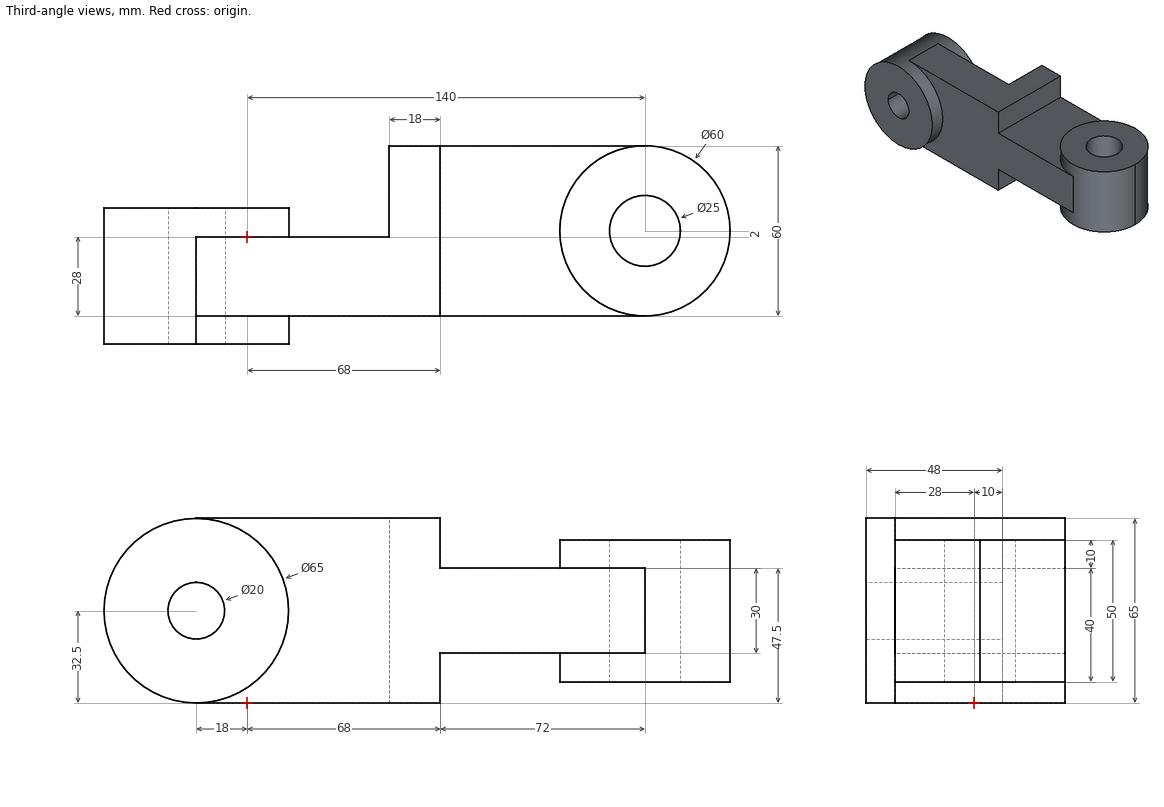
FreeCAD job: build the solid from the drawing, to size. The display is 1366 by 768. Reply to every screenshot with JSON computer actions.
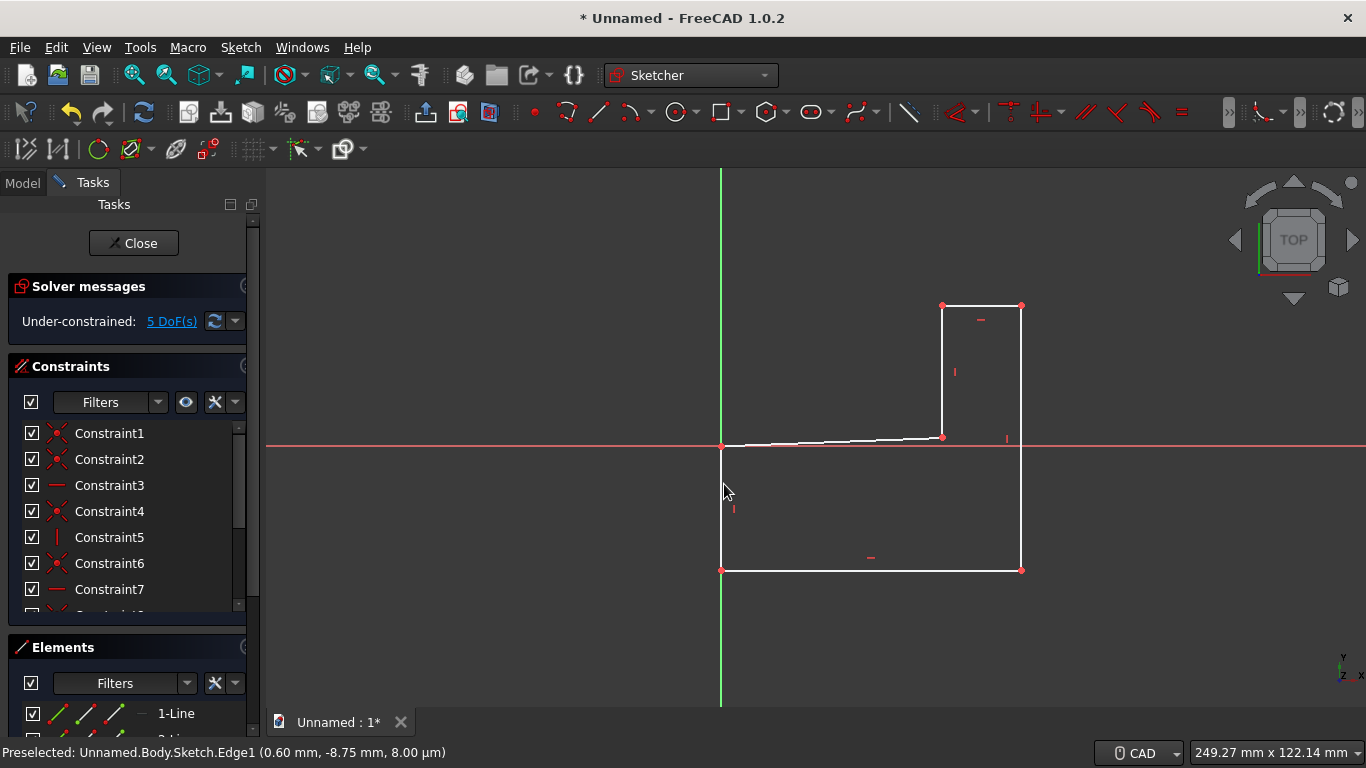
{"action": "left_click", "coordinate": [788, 444]}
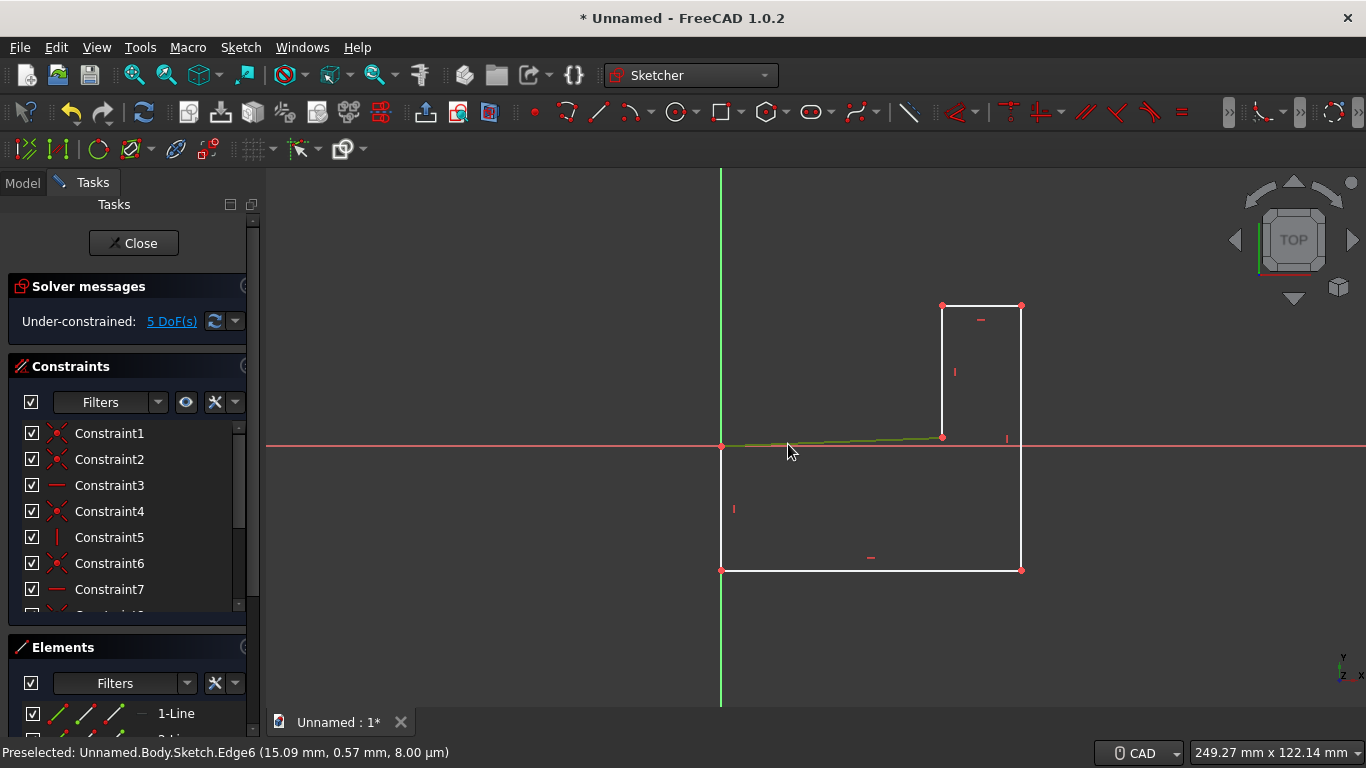
{"action": "key", "text": "h"}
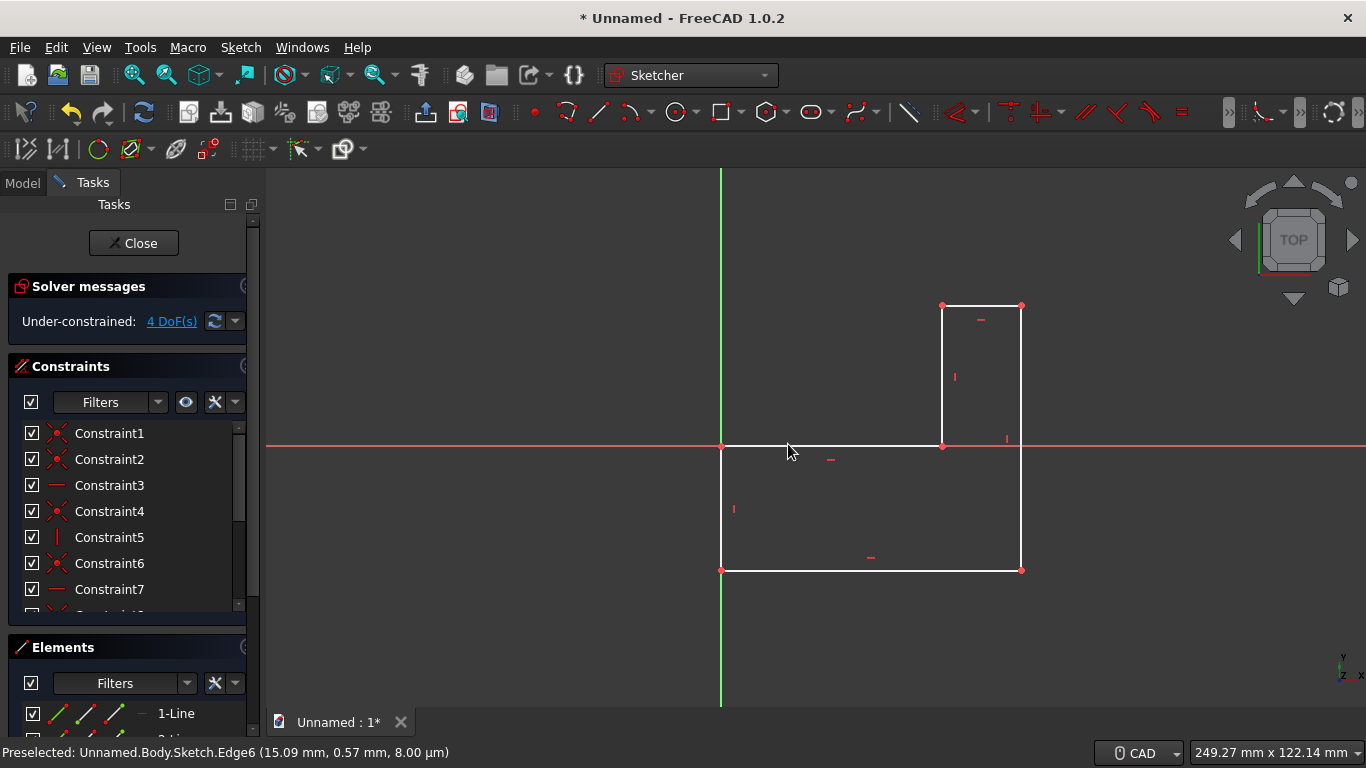
{"action": "key", "text": "d"}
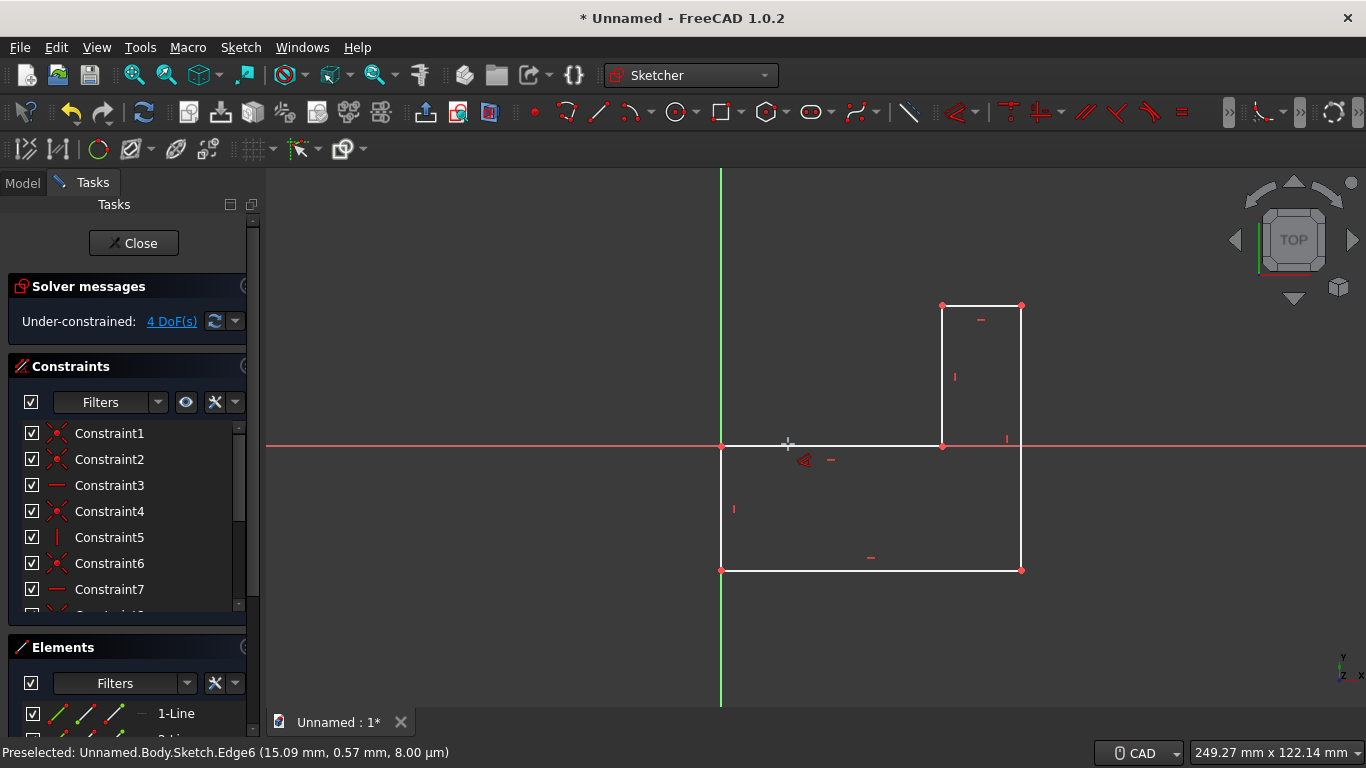
{"action": "left_click", "coordinate": [721, 484]}
{"action": "left_click", "coordinate": [687, 509]}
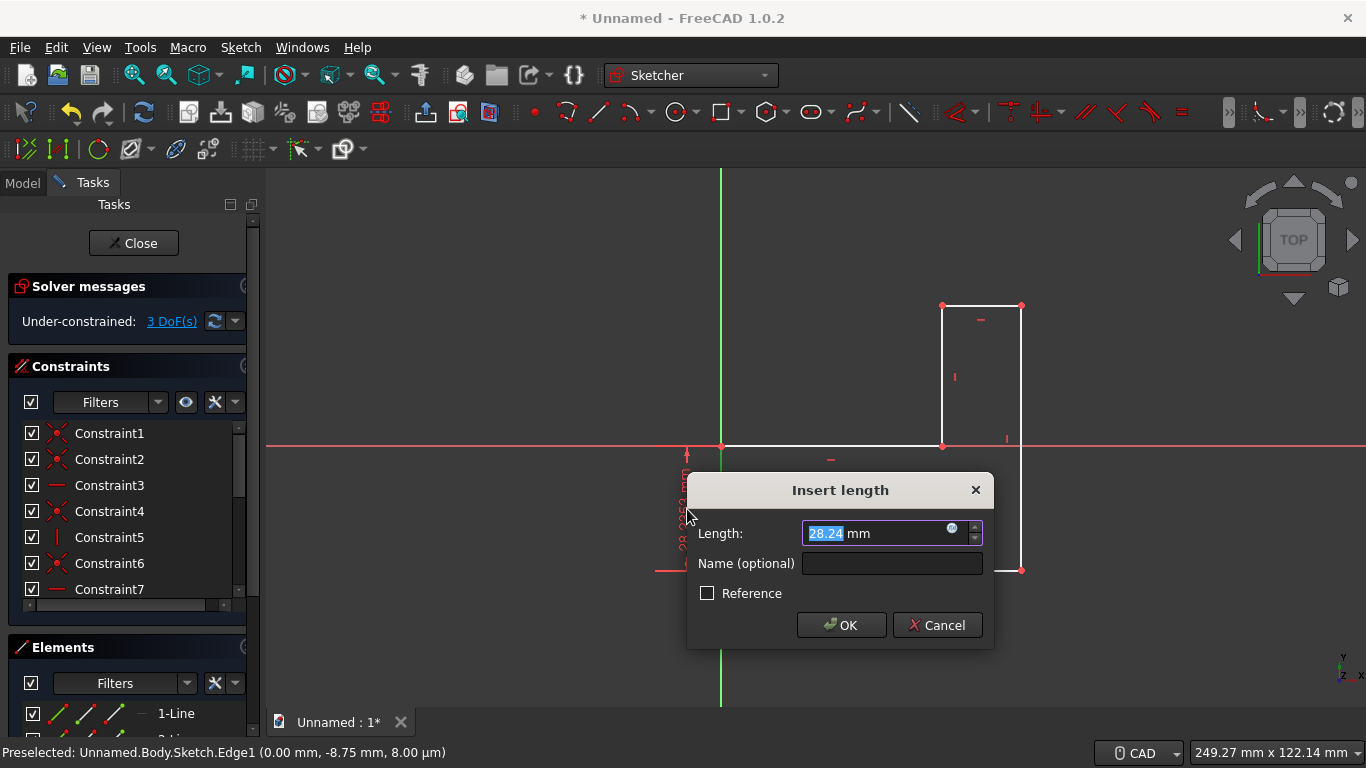
{"action": "type", "text": "28"}
{"action": "key", "text": "Return"}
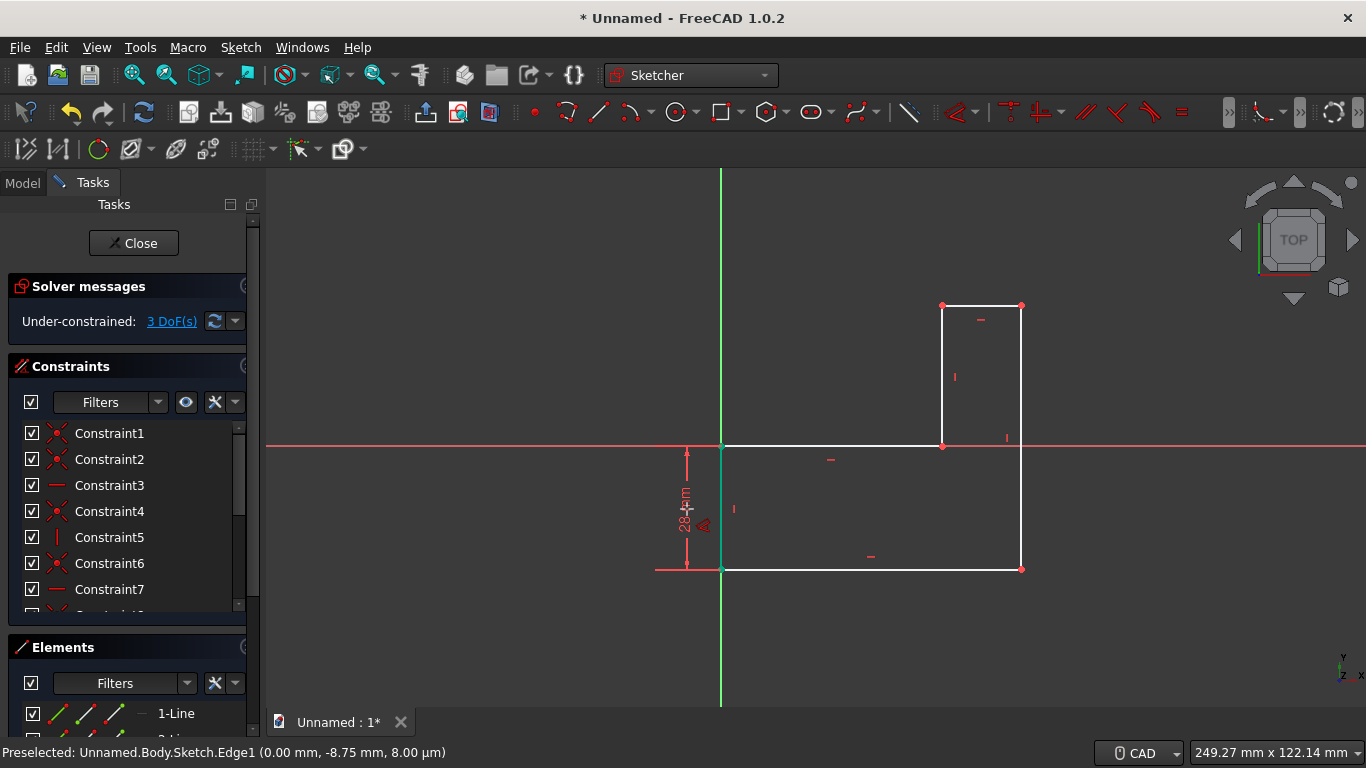
{"action": "left_click", "coordinate": [811, 570]}
{"action": "left_click", "coordinate": [871, 604]}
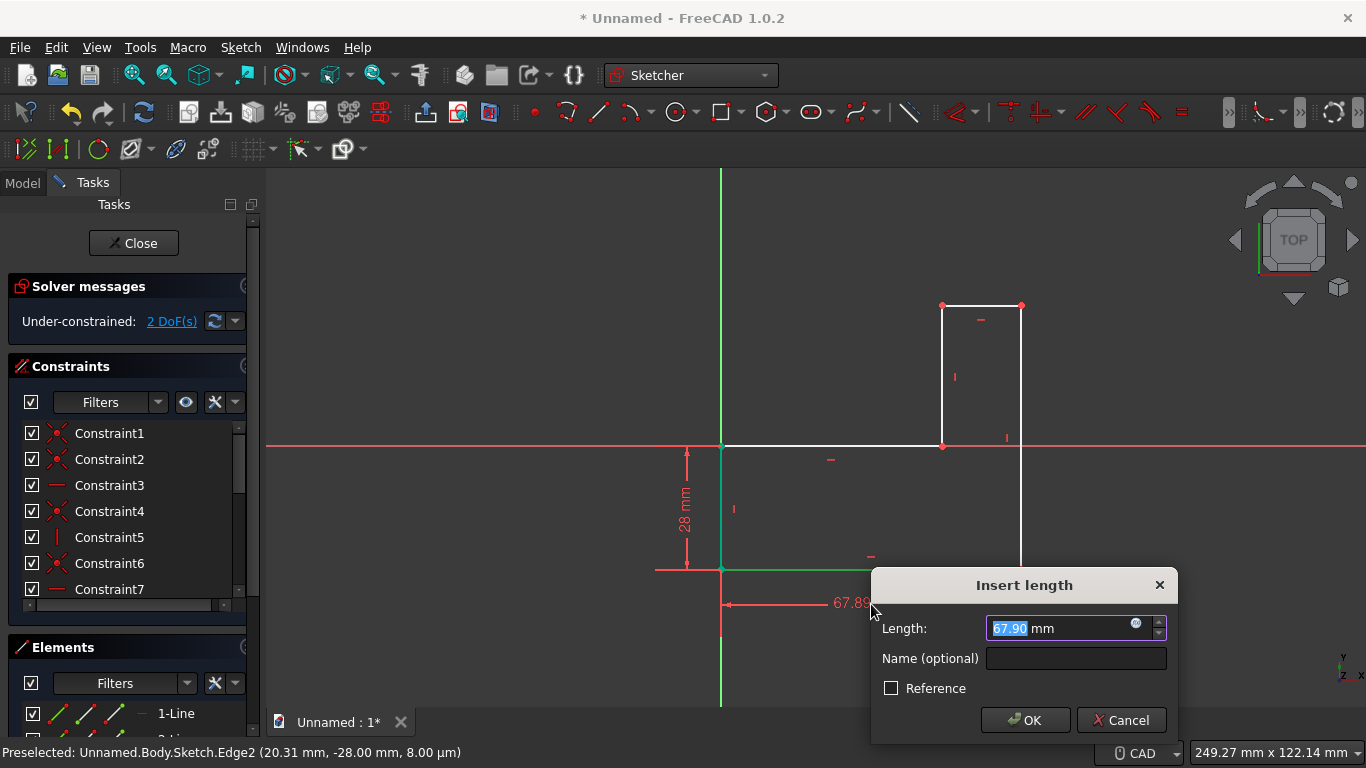
{"action": "type", "text": "68"}
{"action": "key", "text": "Return"}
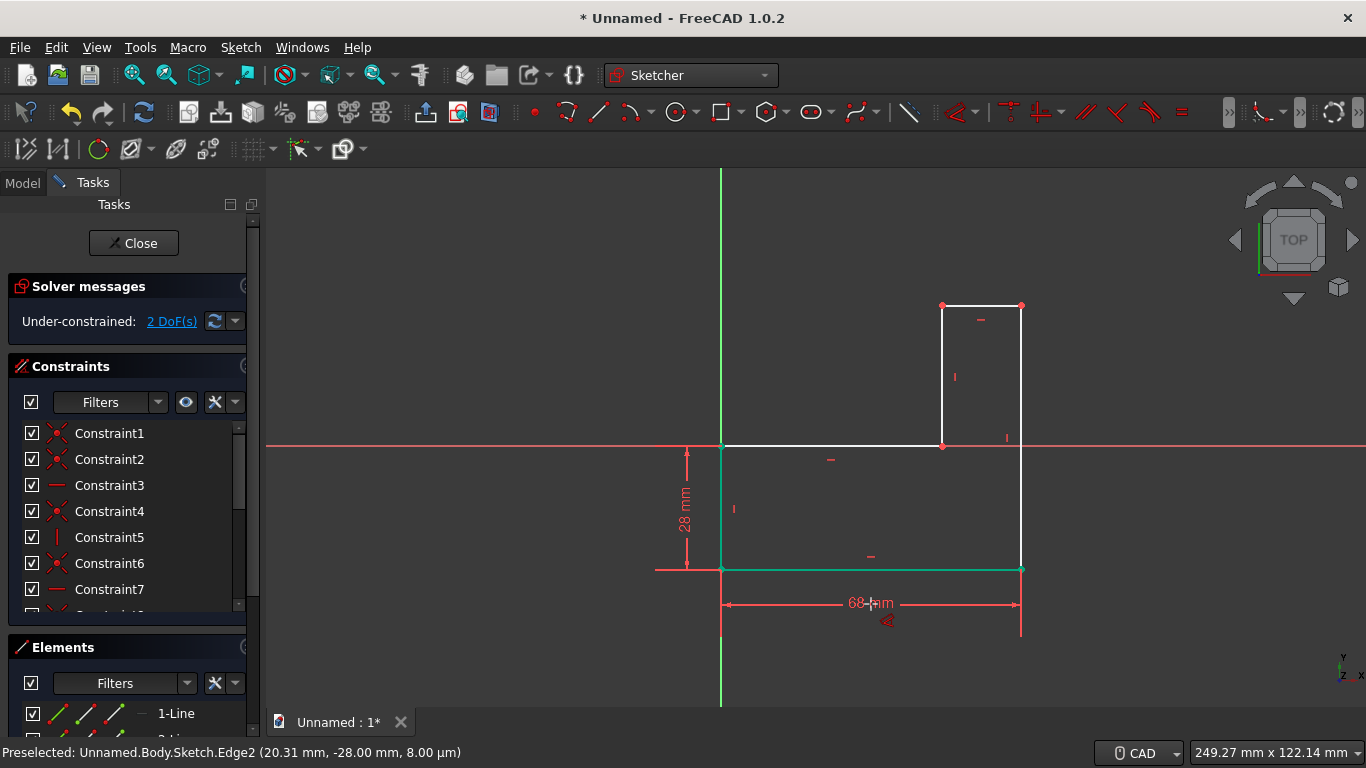
{"action": "left_click", "coordinate": [1021, 491]}
{"action": "left_click", "coordinate": [1055, 377]}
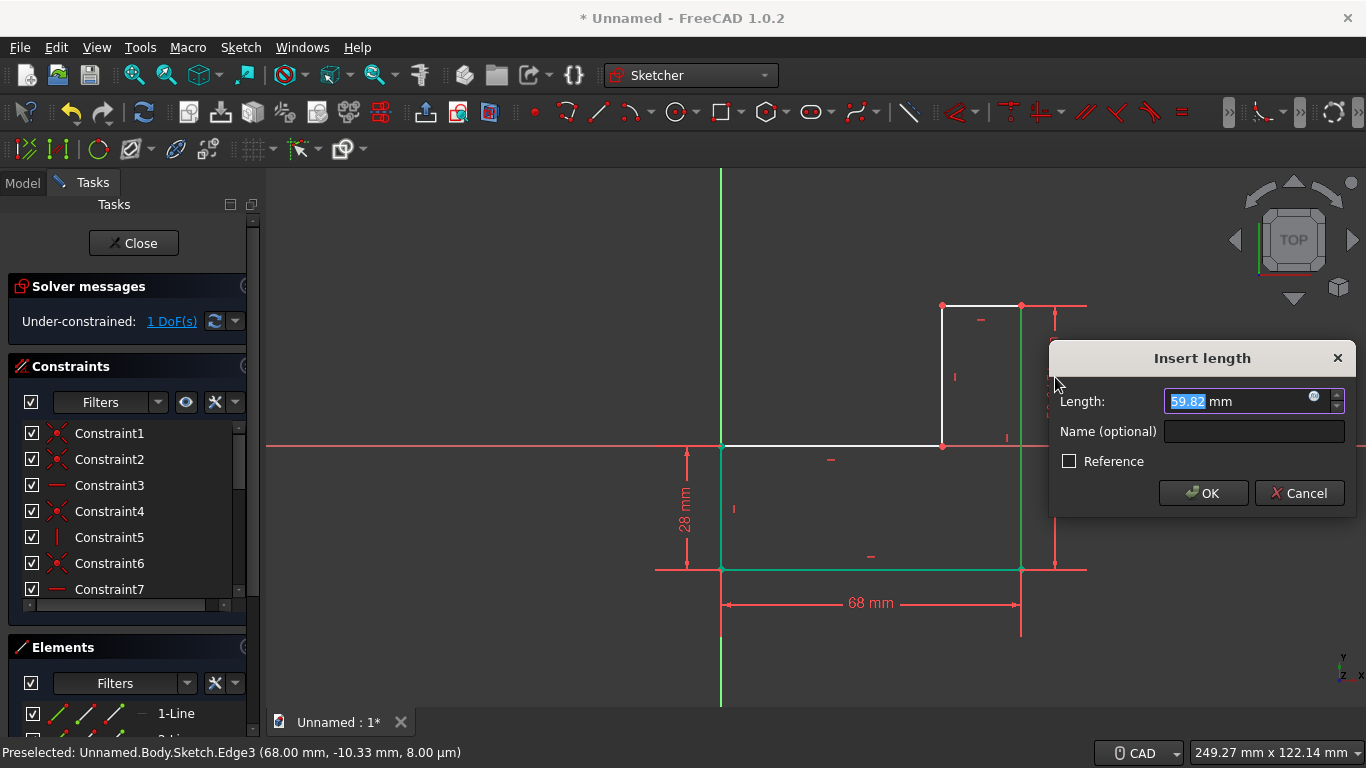
{"action": "type", "text": "60"}
{"action": "key", "text": "Return"}